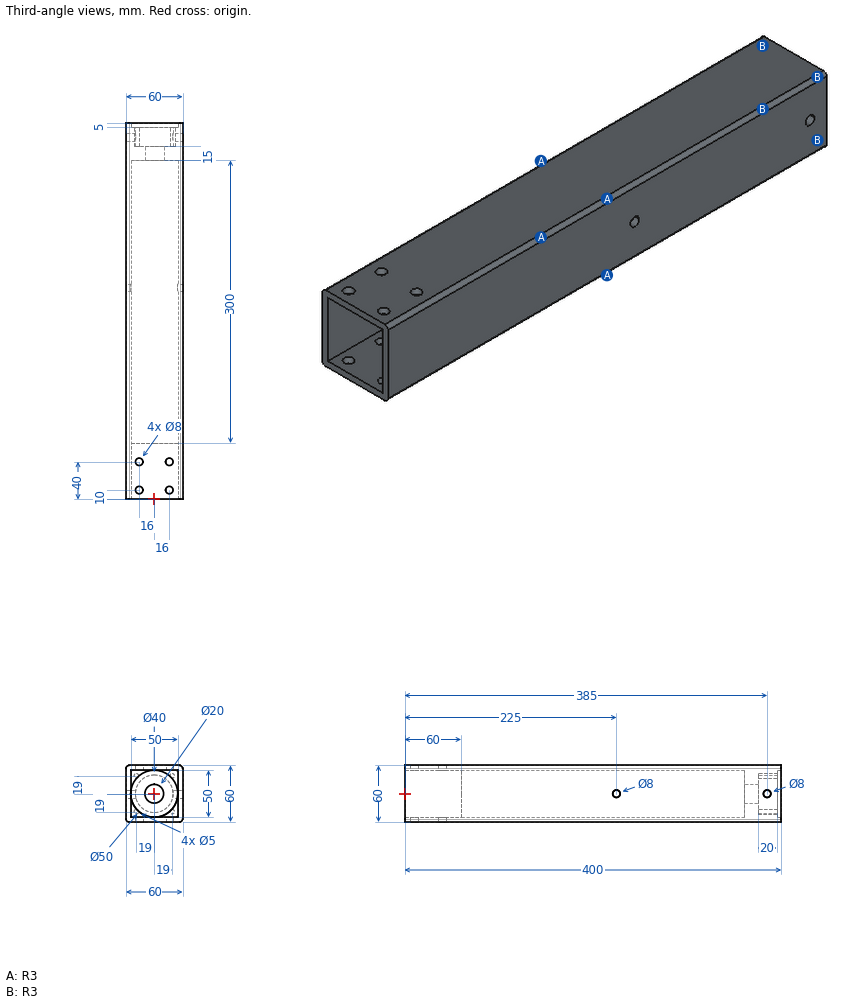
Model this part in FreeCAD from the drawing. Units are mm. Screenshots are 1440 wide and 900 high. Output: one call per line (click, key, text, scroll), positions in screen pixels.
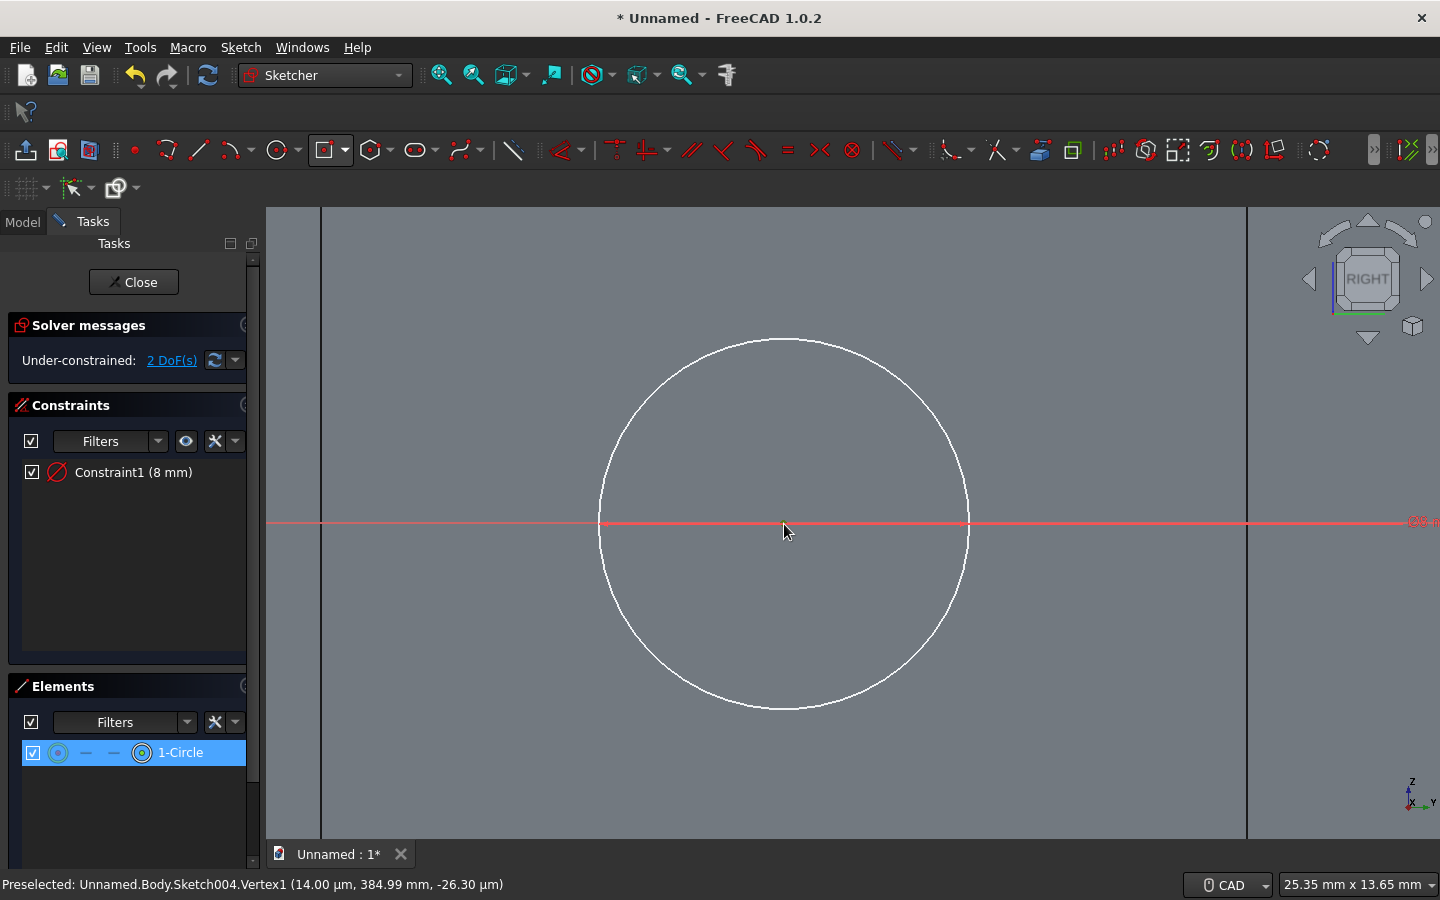
click(364, 523)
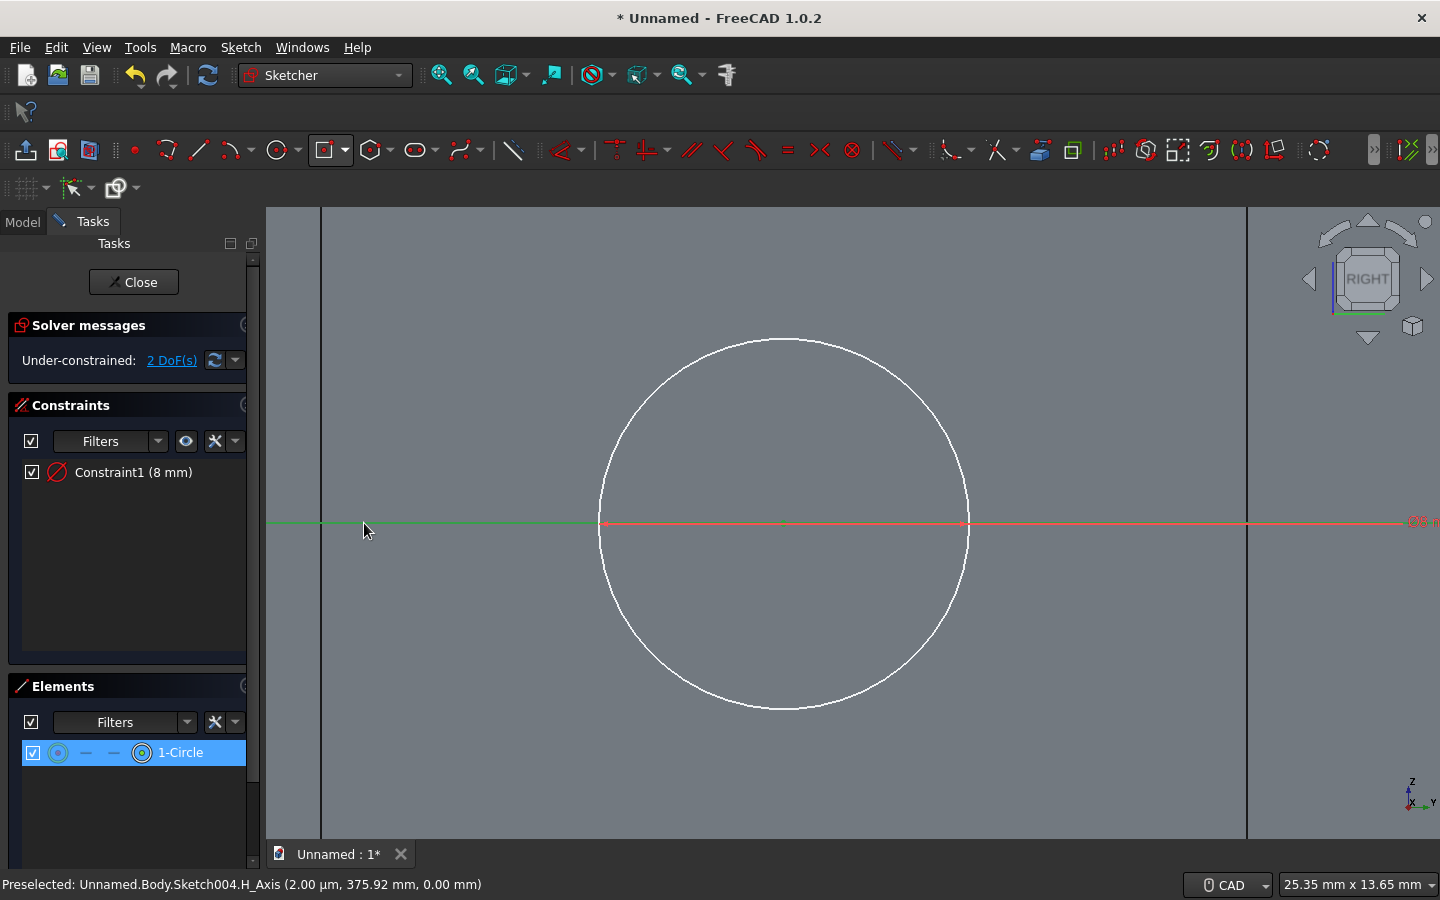
click(616, 150)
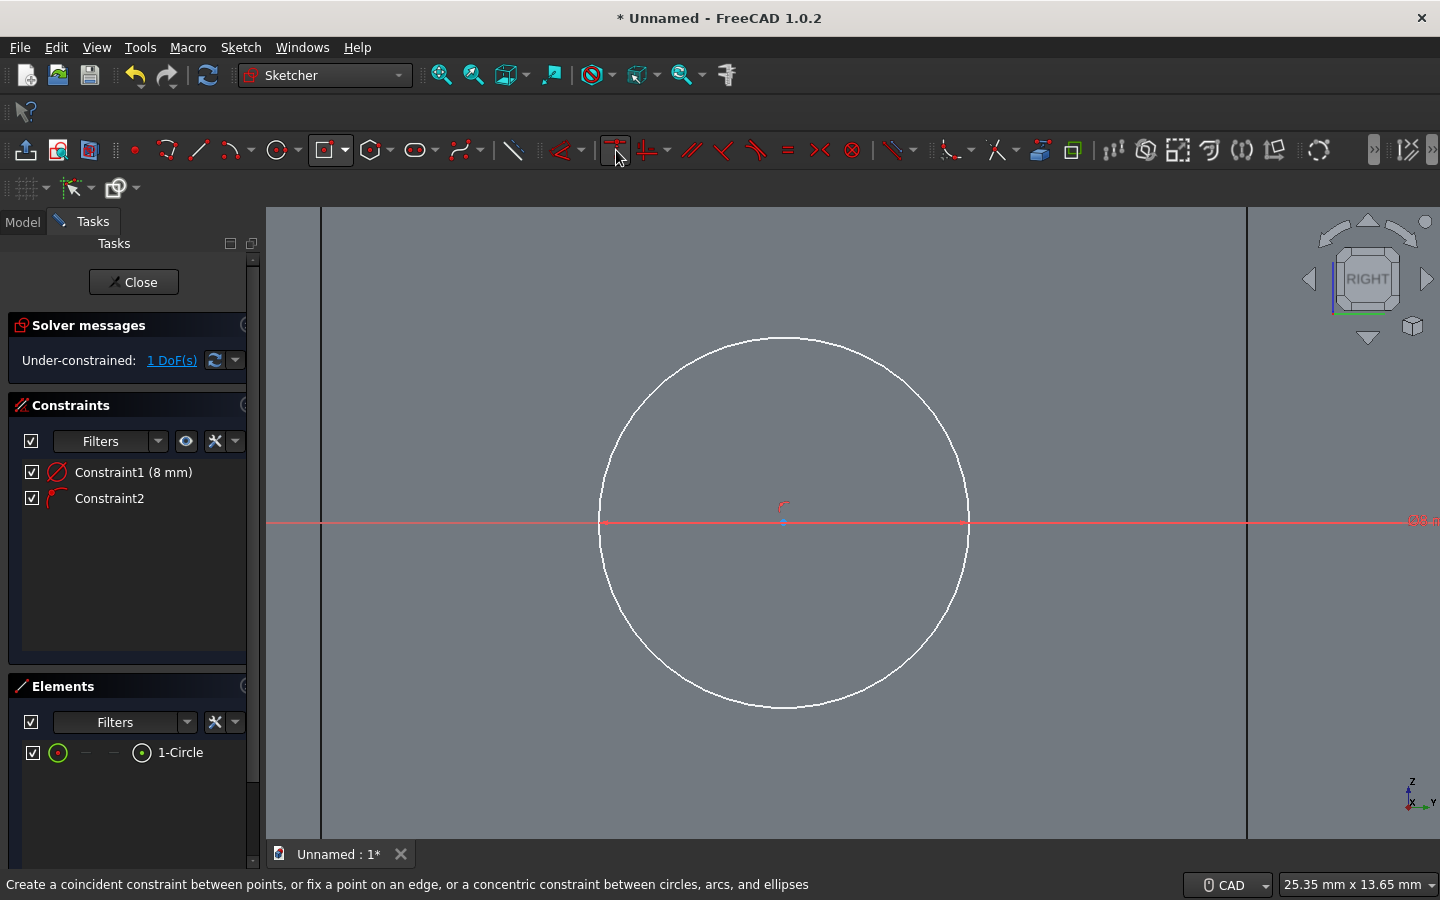
click(560, 150)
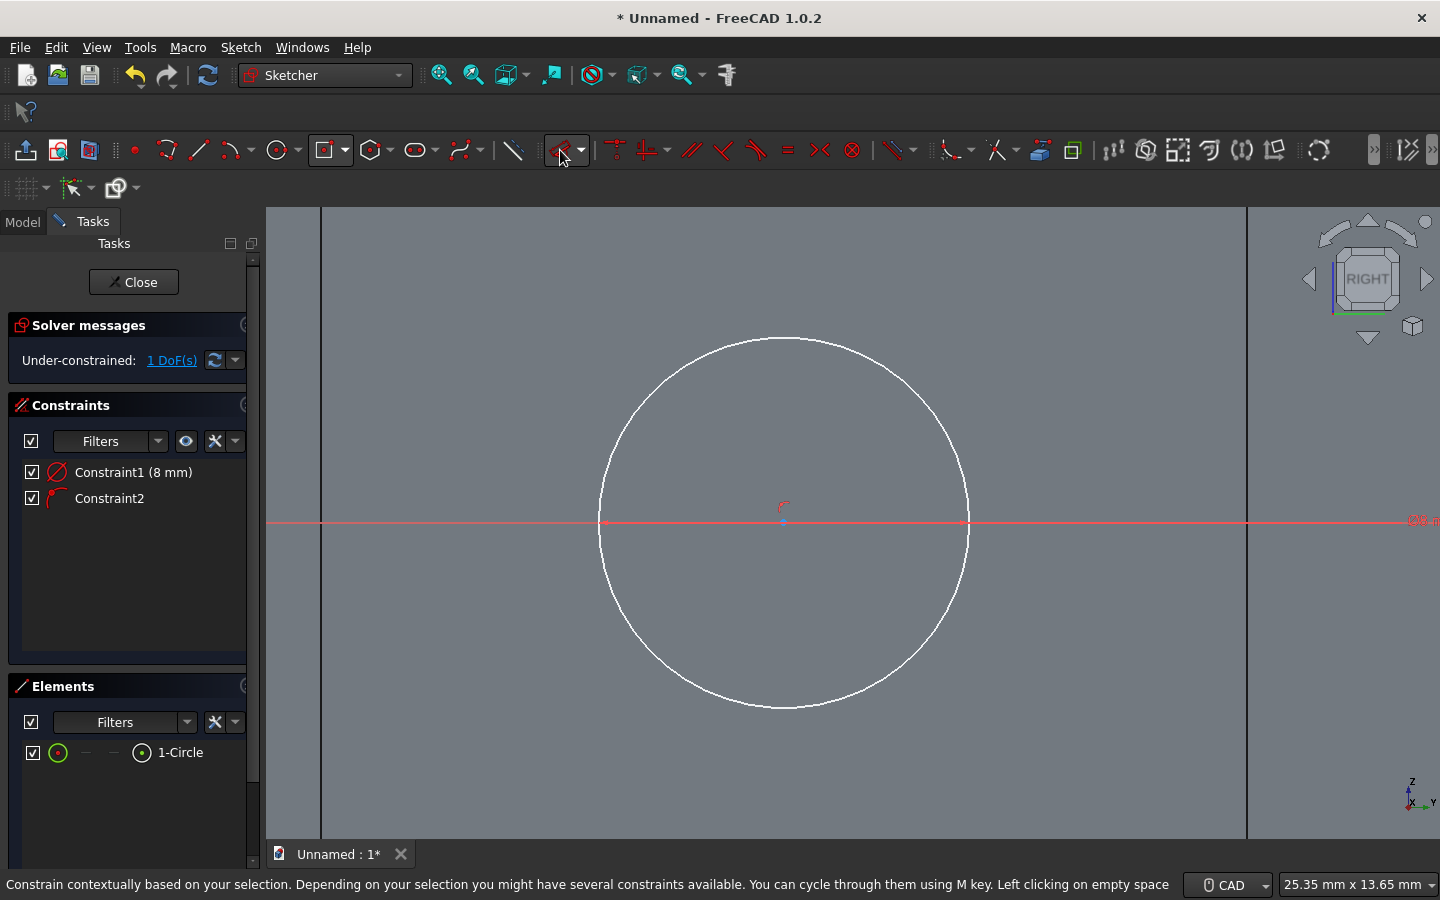
click(784, 523)
click(539, 557)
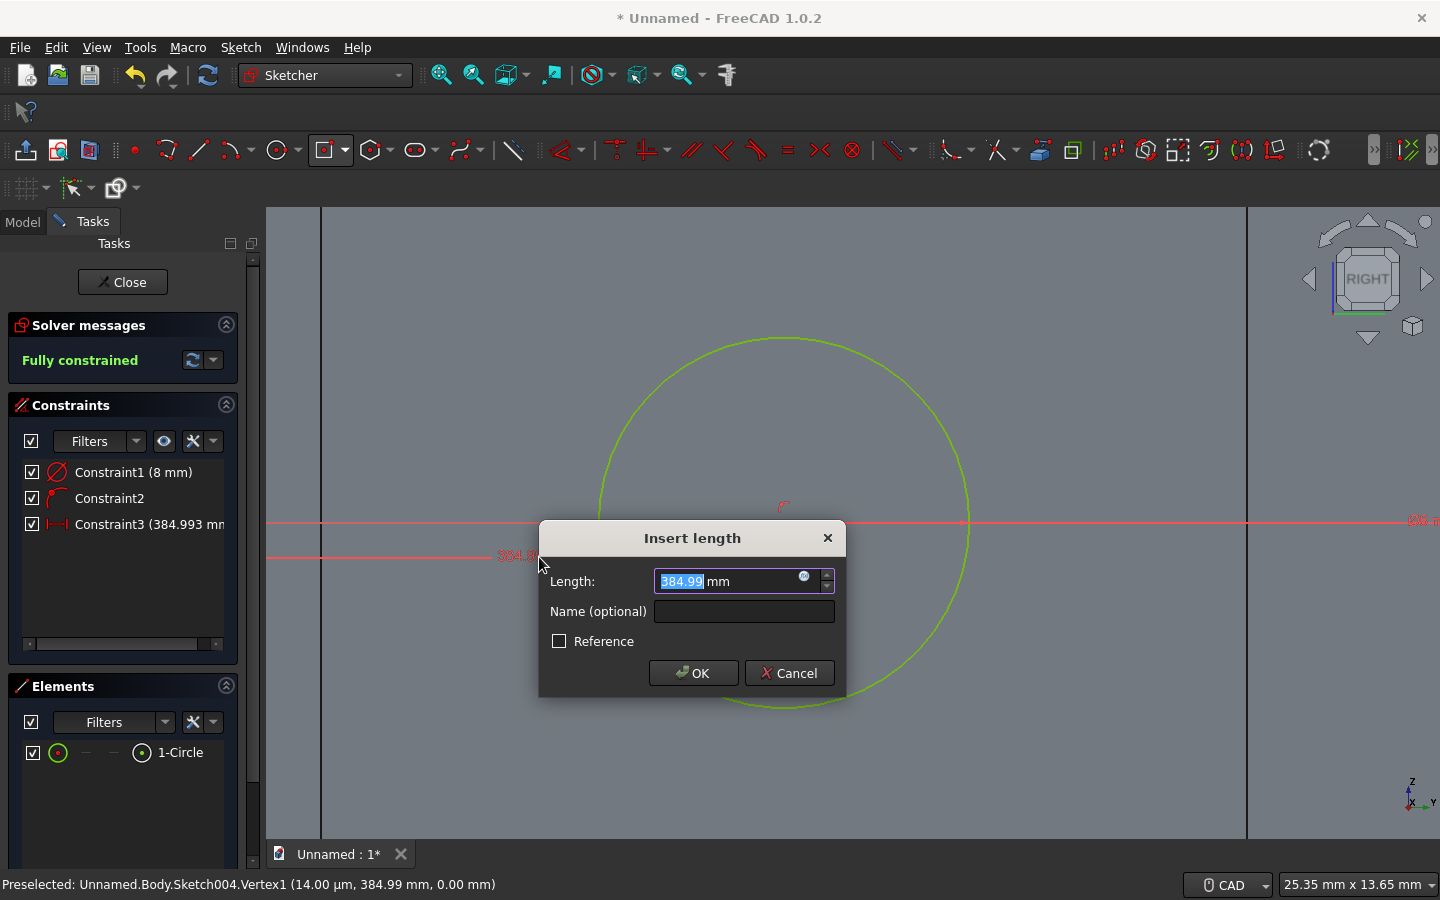
text(385)
key(Return)
key(Escape)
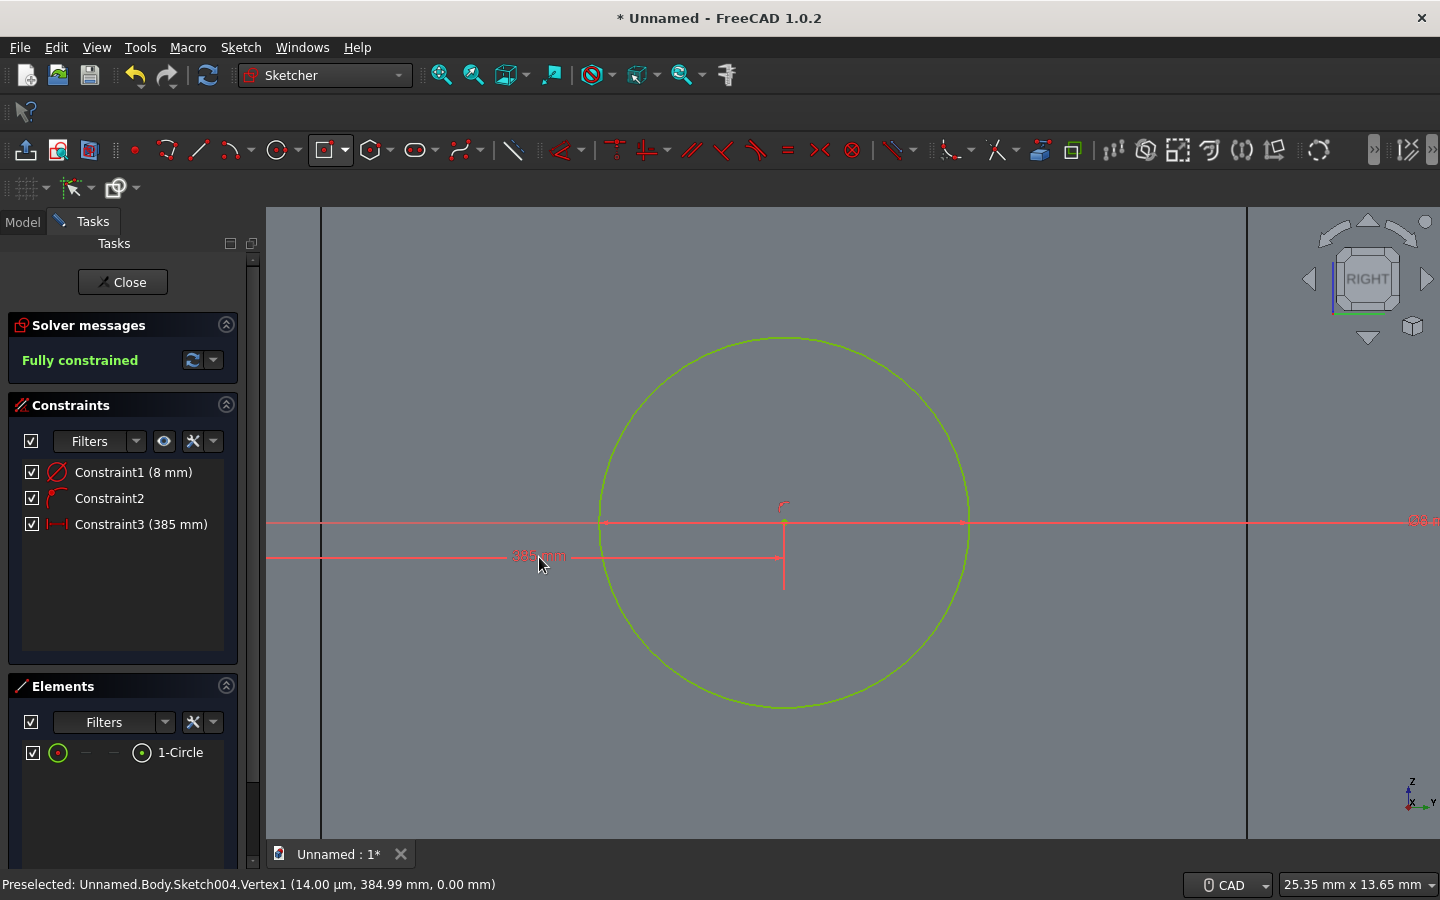
click(123, 282)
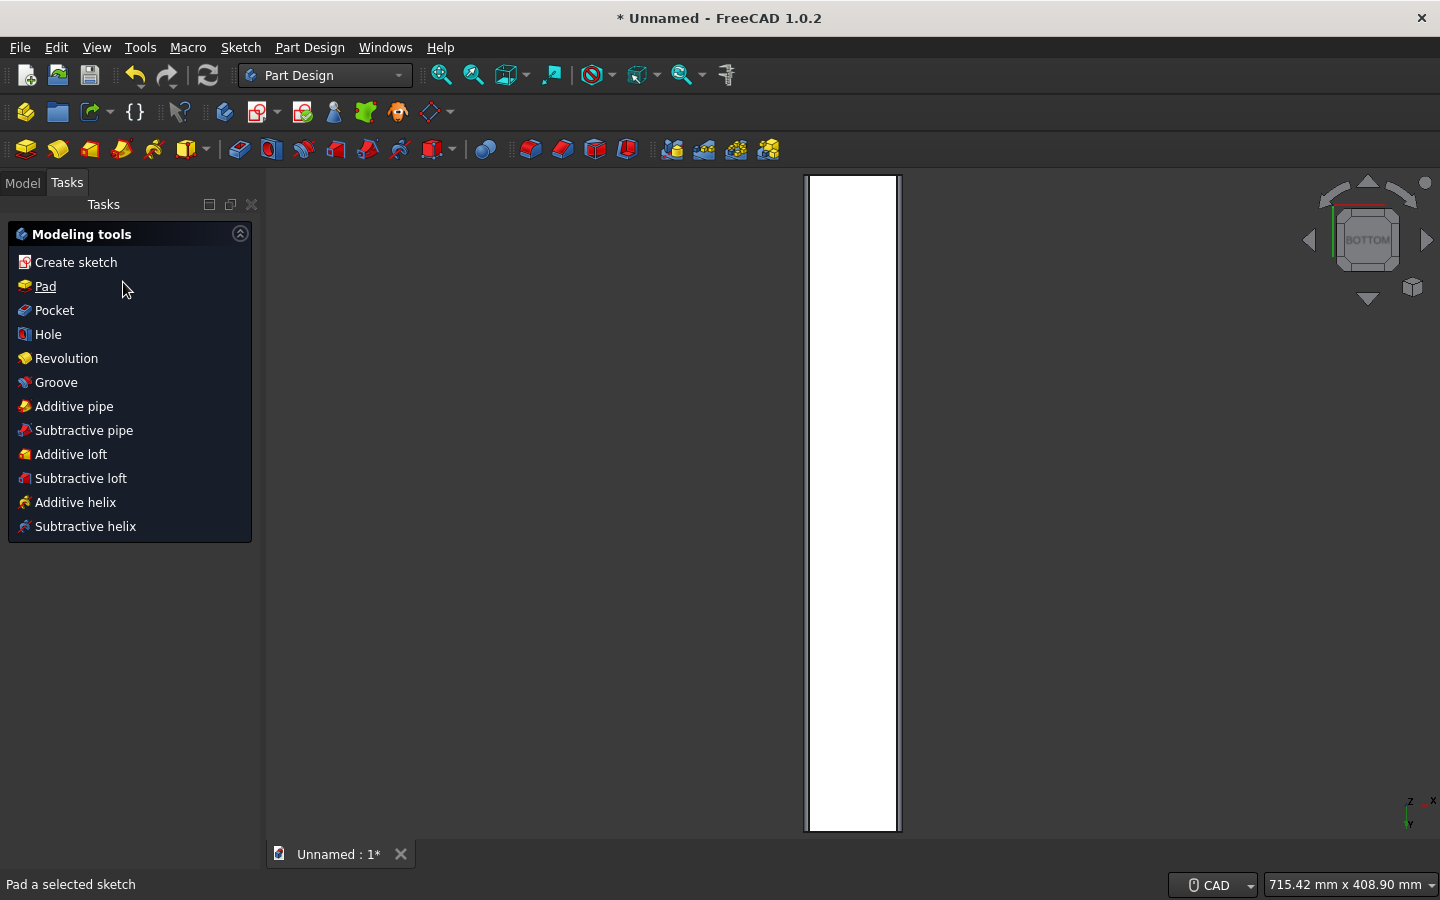
click(240, 150)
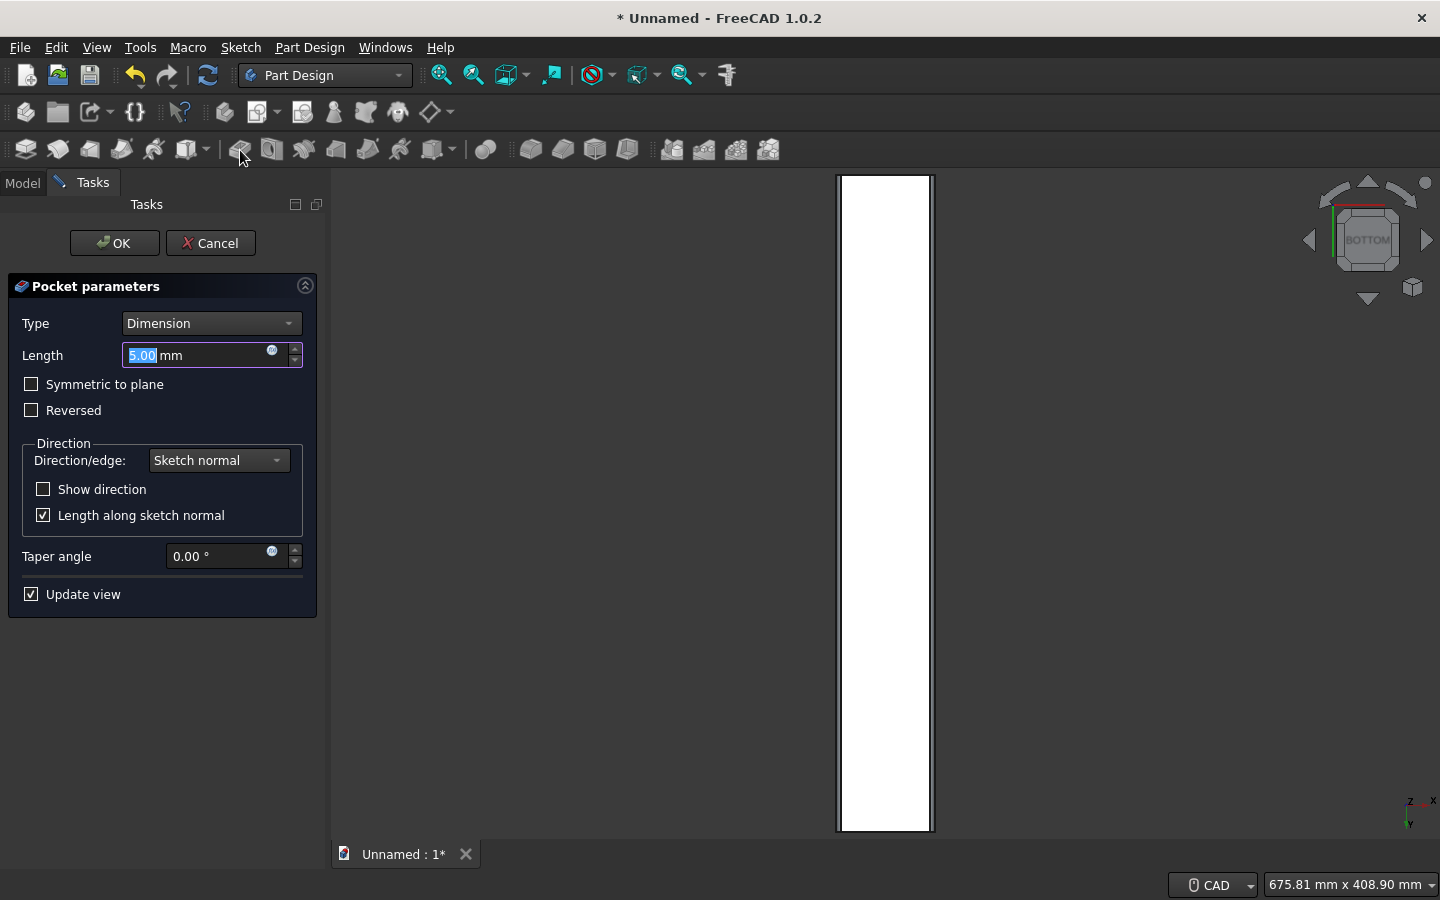
text(60)
key(Tab)